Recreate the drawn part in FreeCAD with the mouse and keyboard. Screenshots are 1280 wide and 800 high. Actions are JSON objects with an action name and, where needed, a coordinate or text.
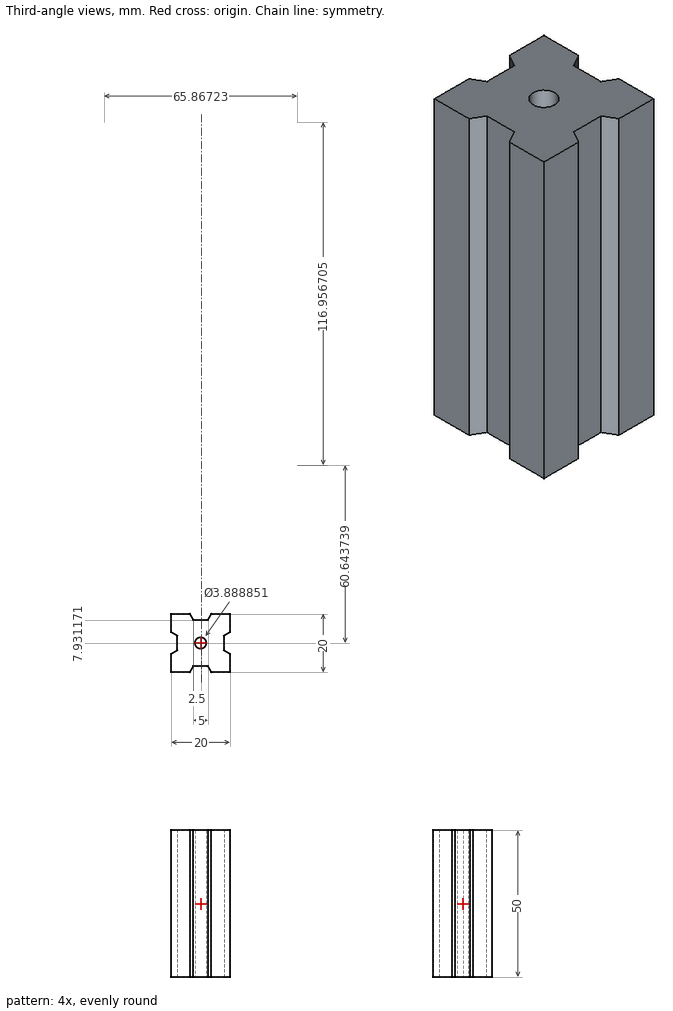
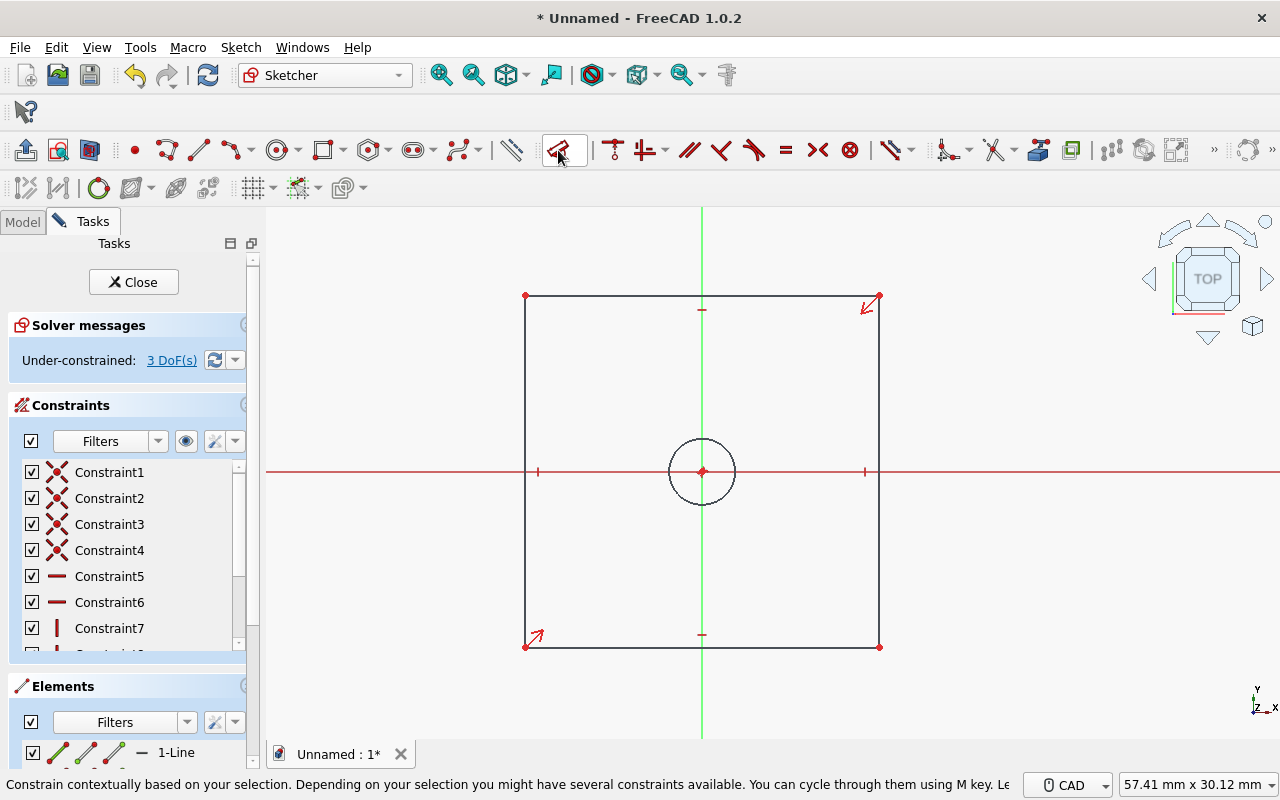
{"action": "left_click", "coordinate": [725, 448]}
{"action": "left_click", "coordinate": [747, 425]}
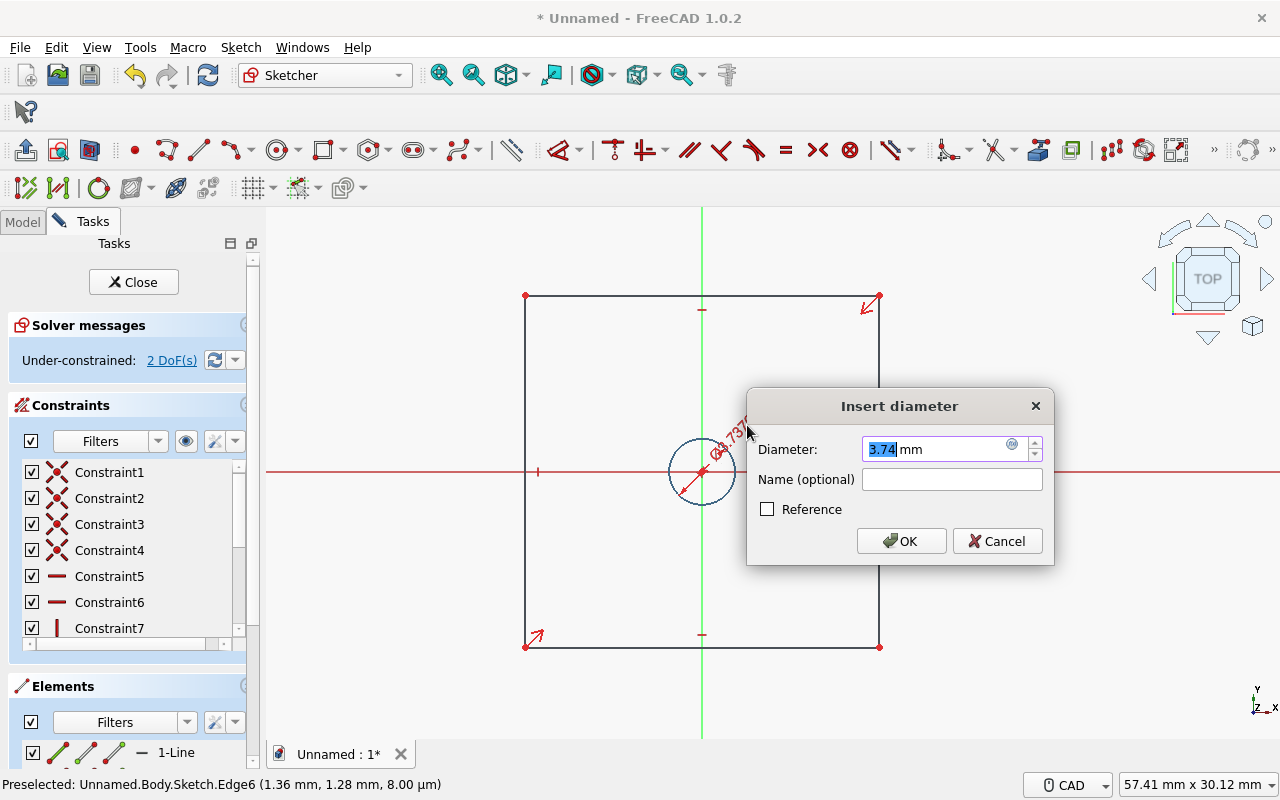
{"action": "type", "text": "3.888851"}
{"action": "key", "text": "Return"}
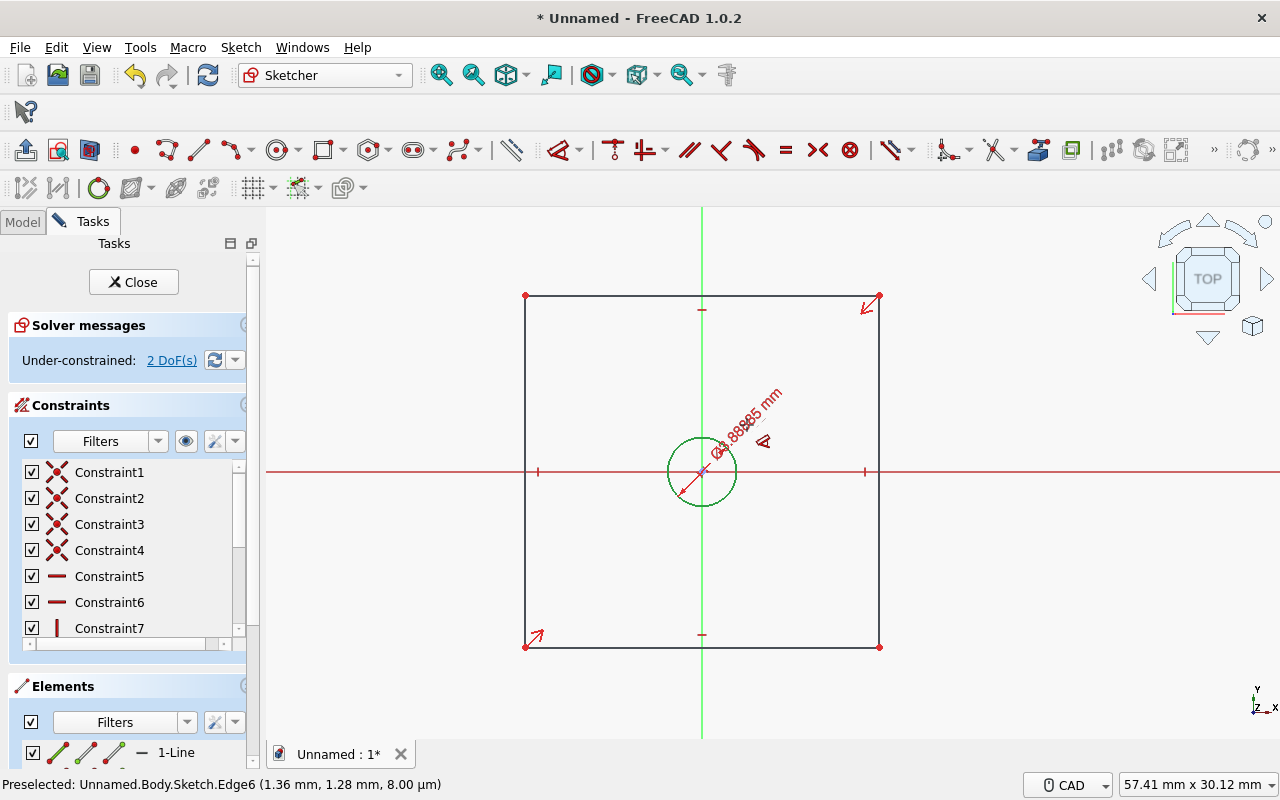
{"action": "left_click", "coordinate": [631, 648]}
{"action": "left_click", "coordinate": [621, 682]}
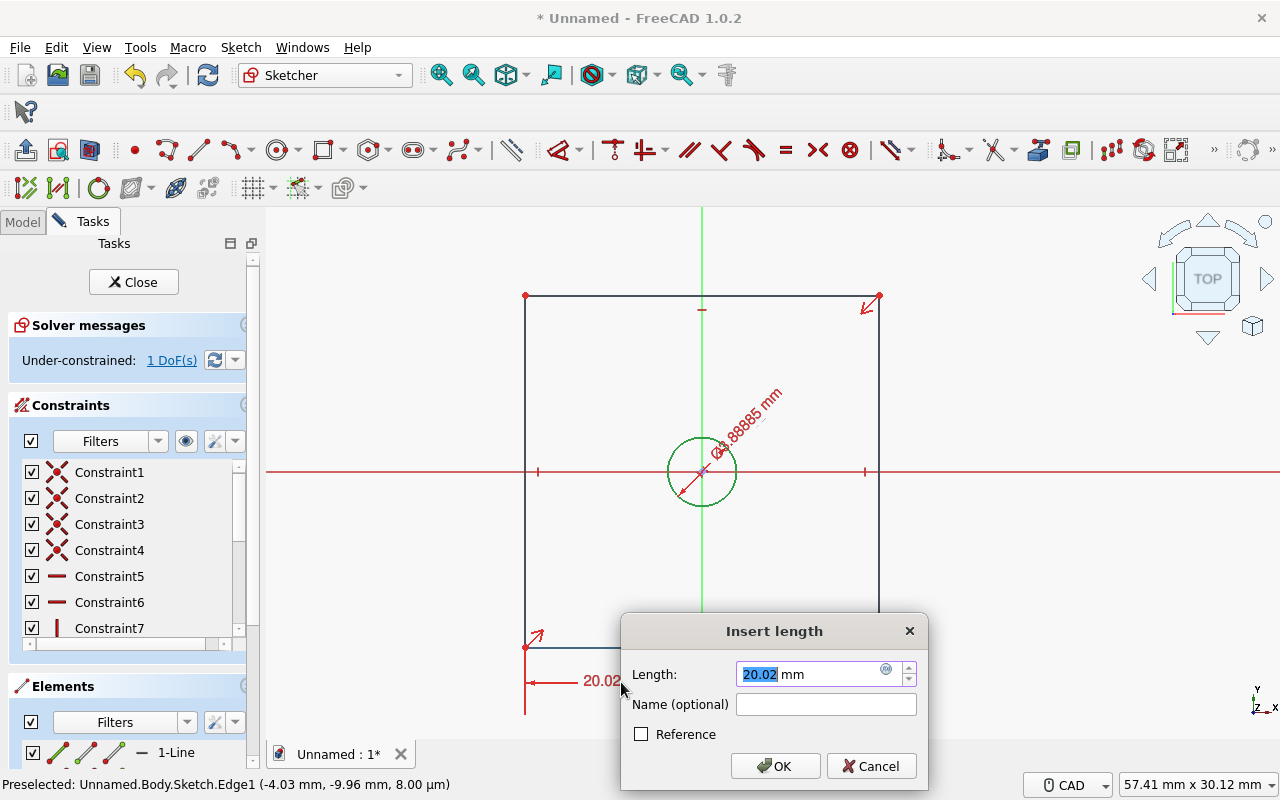
{"action": "type", "text": "20"}
{"action": "key", "text": "Return"}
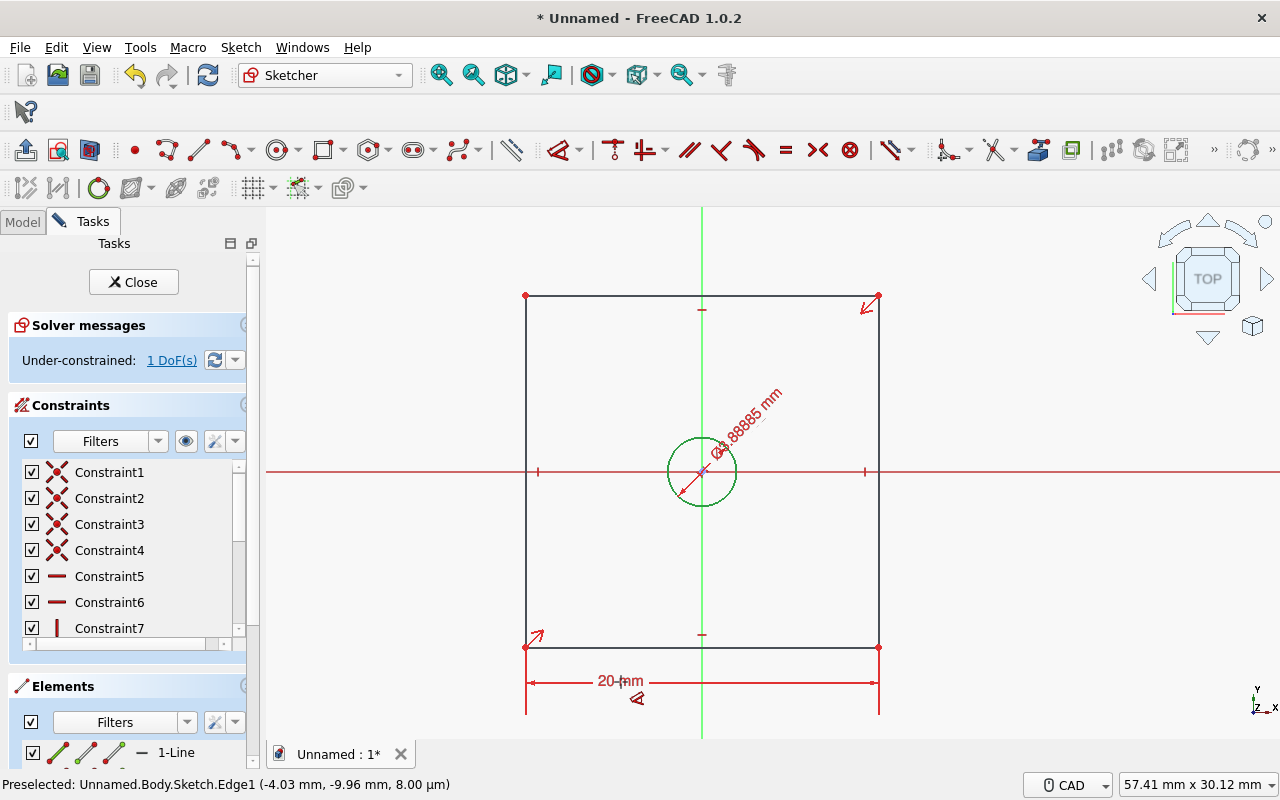
{"action": "left_click", "coordinate": [879, 542]}
{"action": "left_click", "coordinate": [913, 391]}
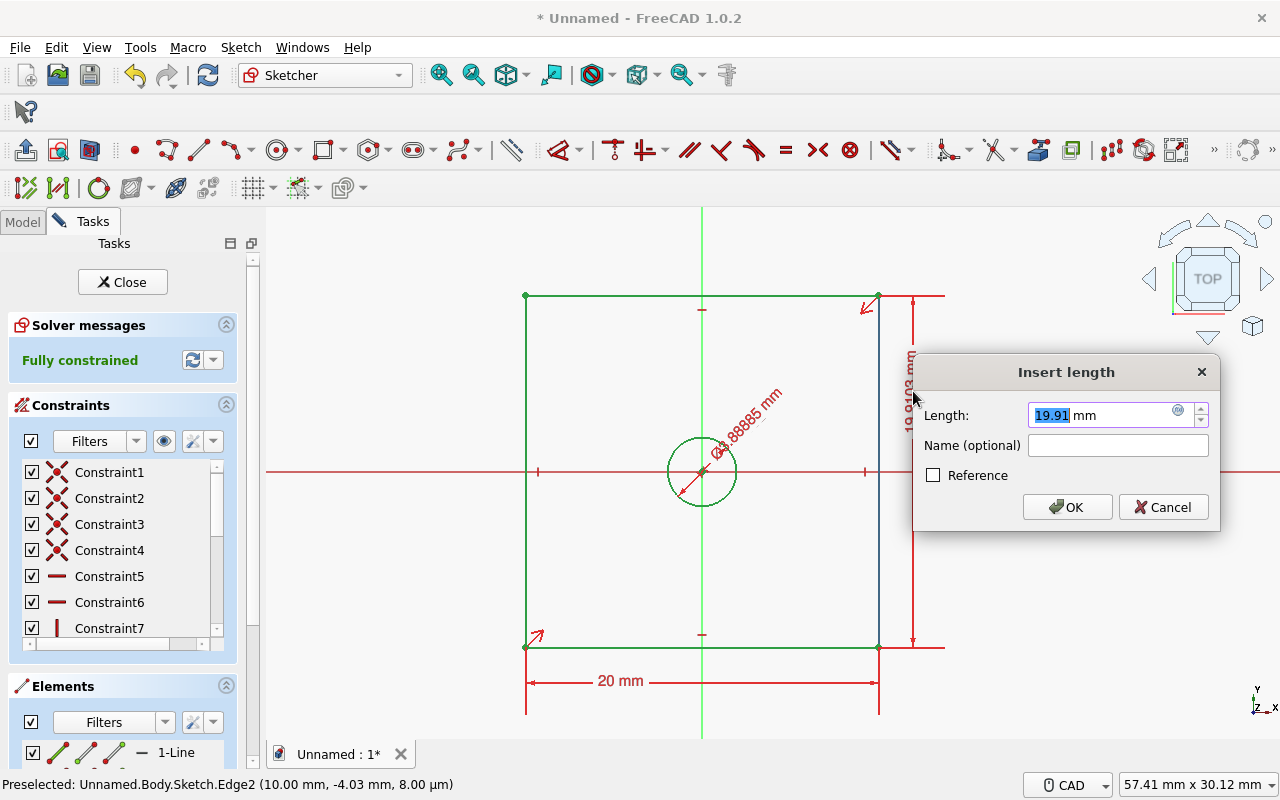
{"action": "type", "text": "20"}
{"action": "key", "text": "Return"}
{"action": "key", "text": "Escape"}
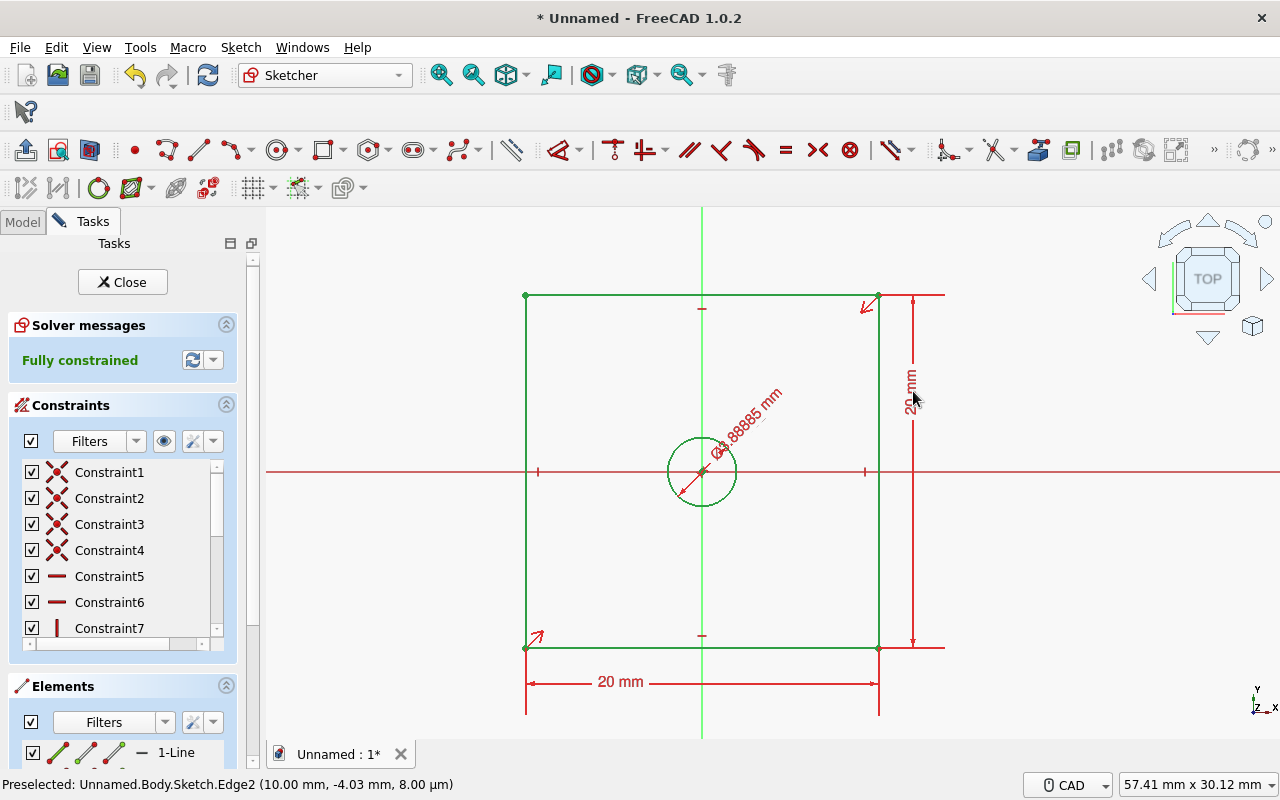
{"action": "left_click", "coordinate": [123, 282]}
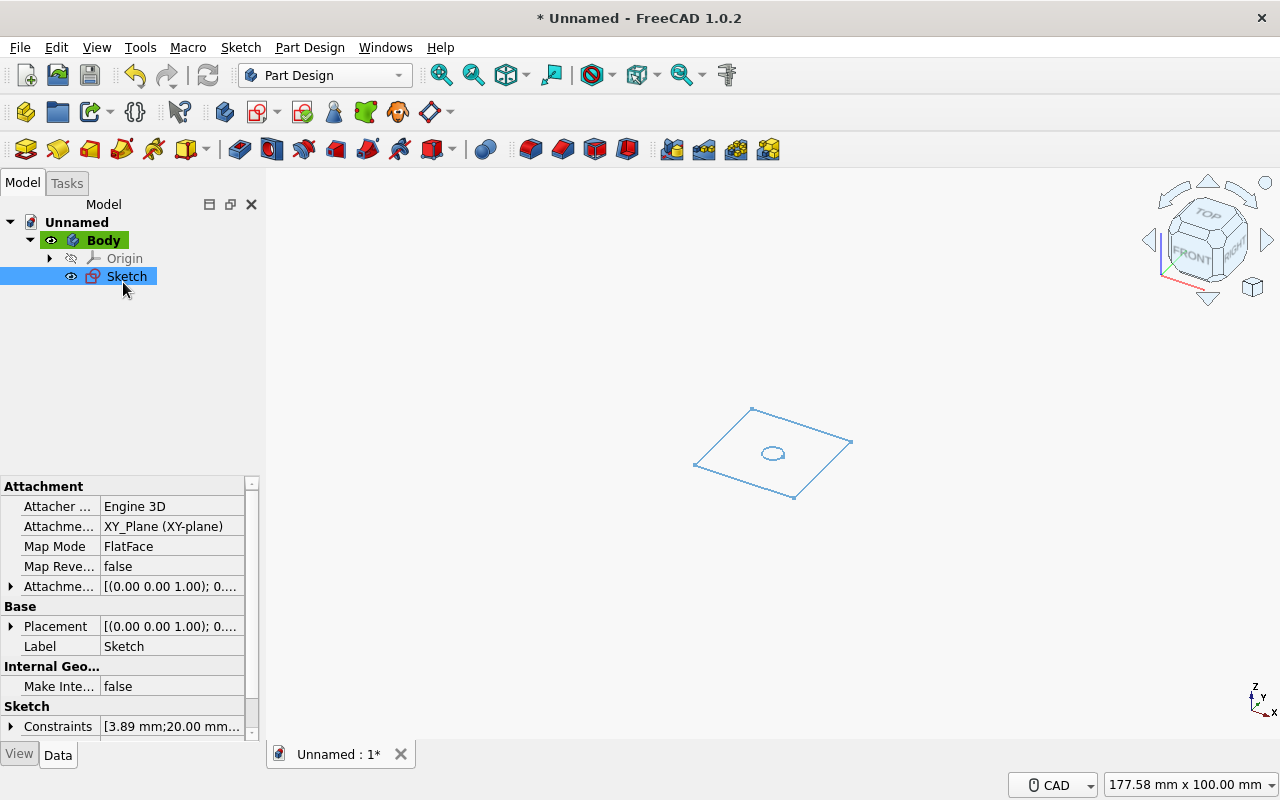
{"action": "left_click", "coordinate": [26, 150]}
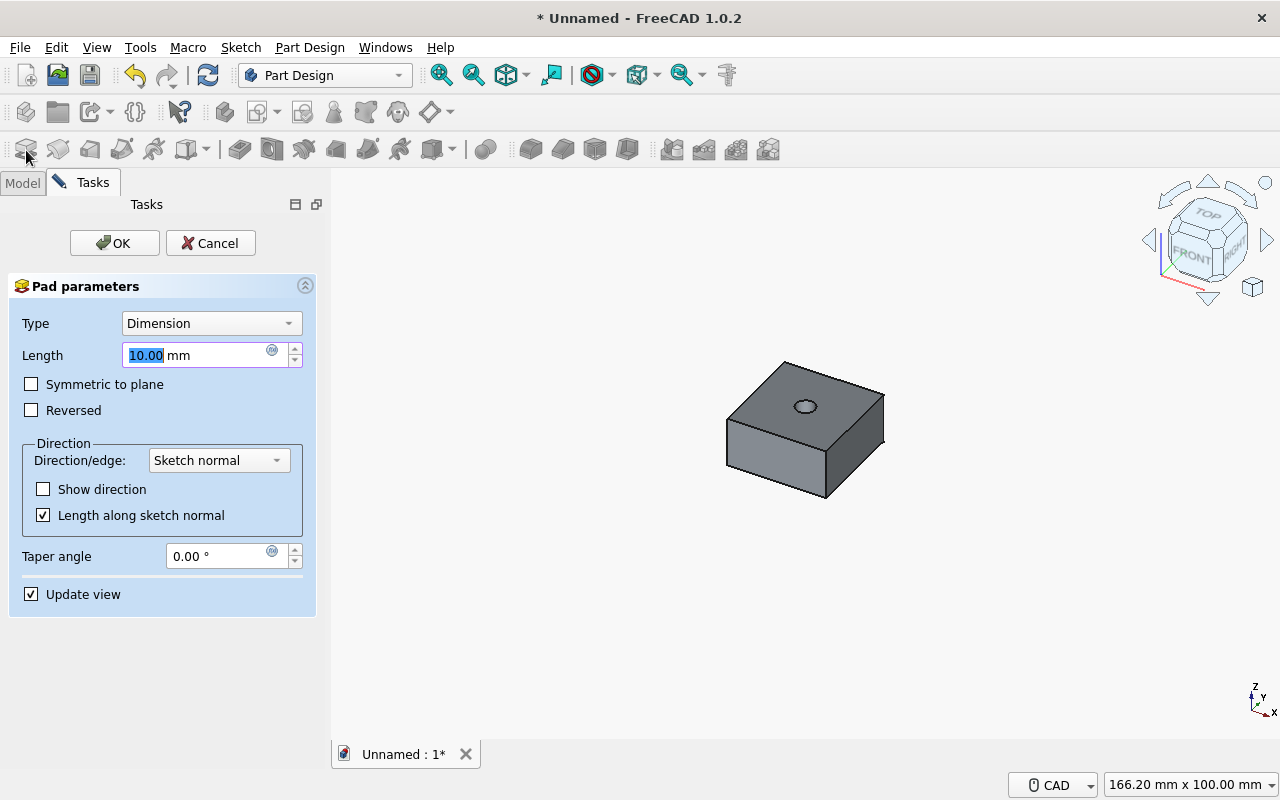
{"action": "type", "text": "50"}
{"action": "key", "text": "Tab"}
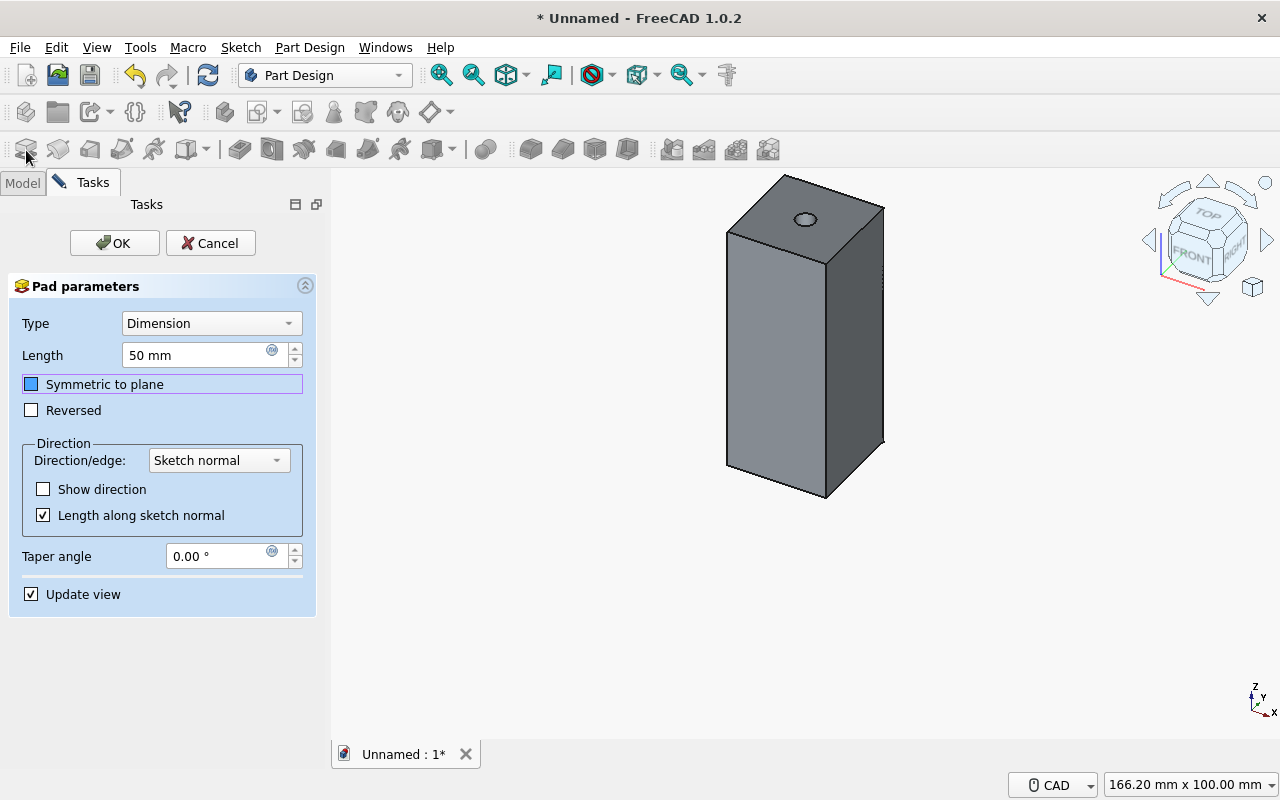
{"action": "left_click", "coordinate": [30, 384]}